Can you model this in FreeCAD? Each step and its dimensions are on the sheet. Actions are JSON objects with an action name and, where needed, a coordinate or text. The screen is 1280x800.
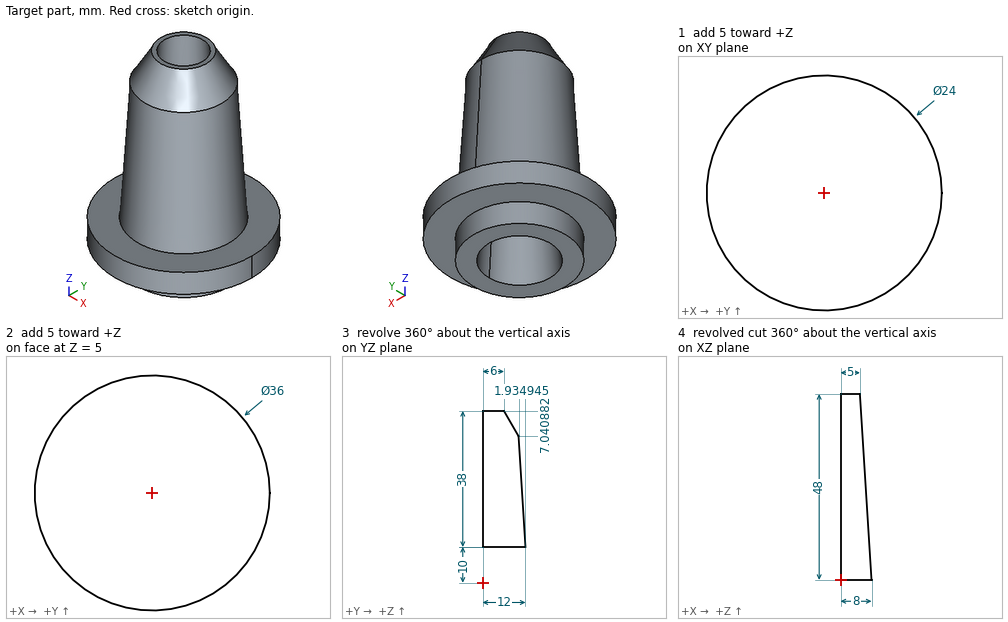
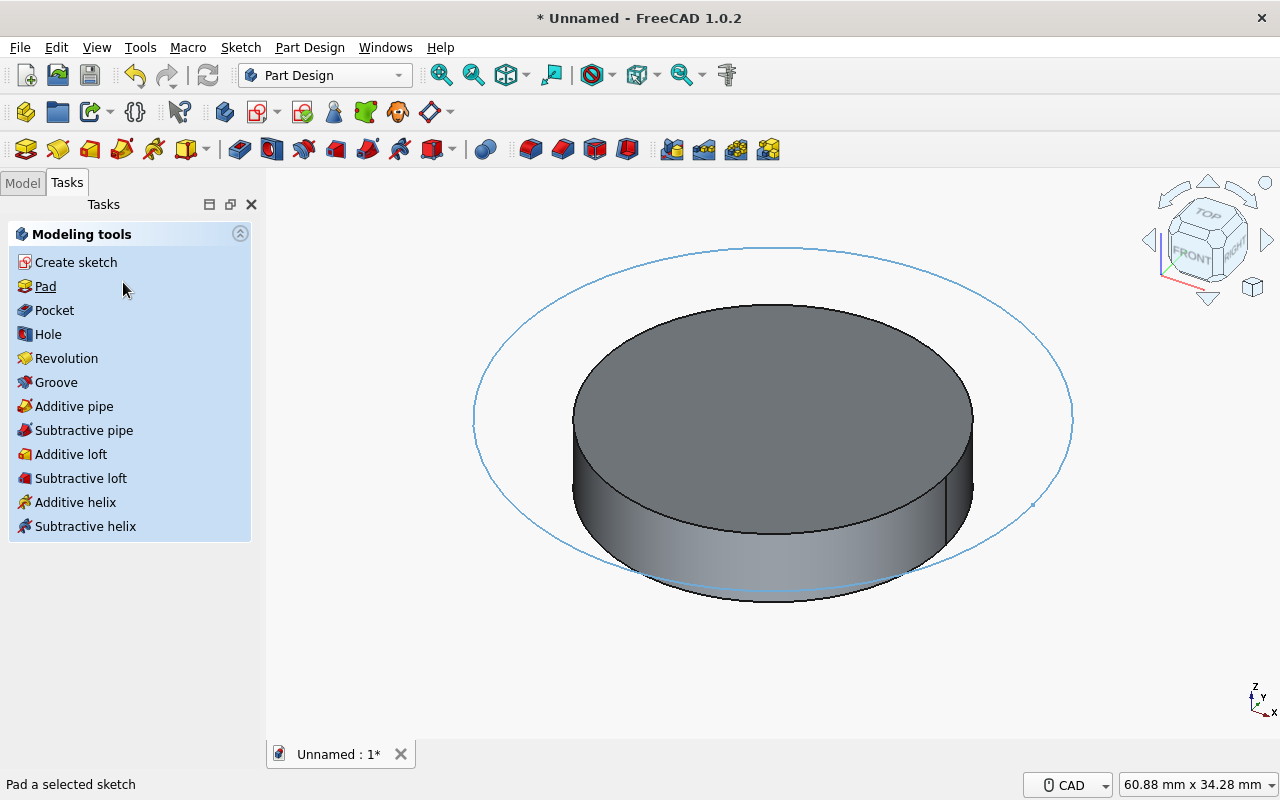
{"action": "left_click", "coordinate": [26, 150]}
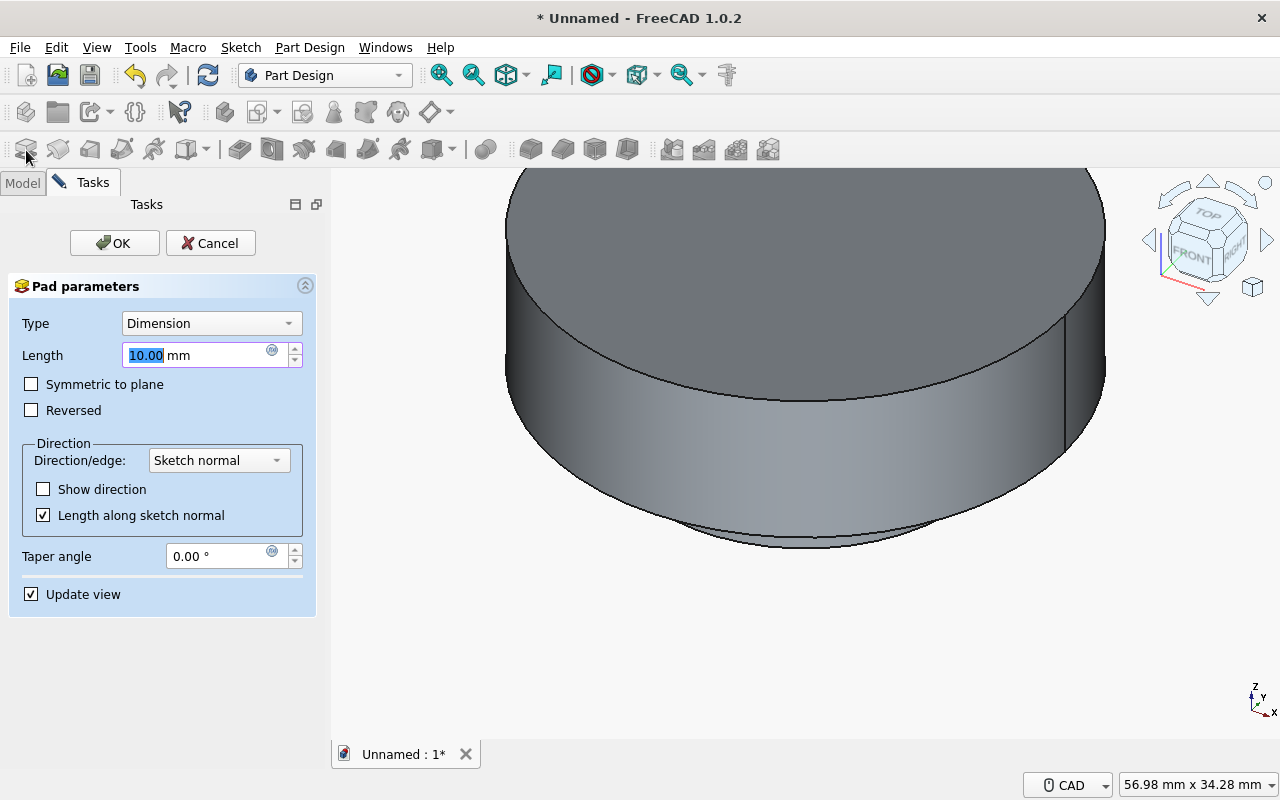
{"action": "type", "text": "5"}
{"action": "key", "text": "Tab"}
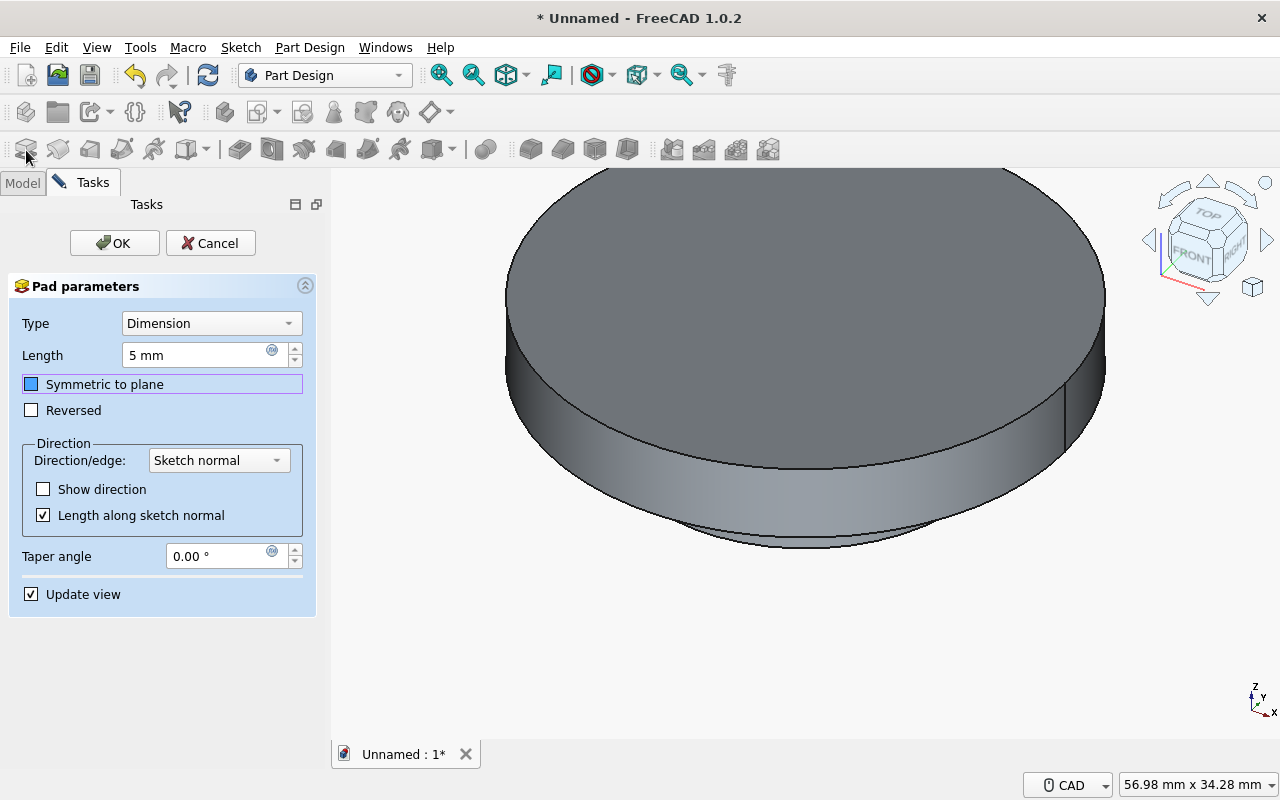
{"action": "left_click", "coordinate": [115, 243]}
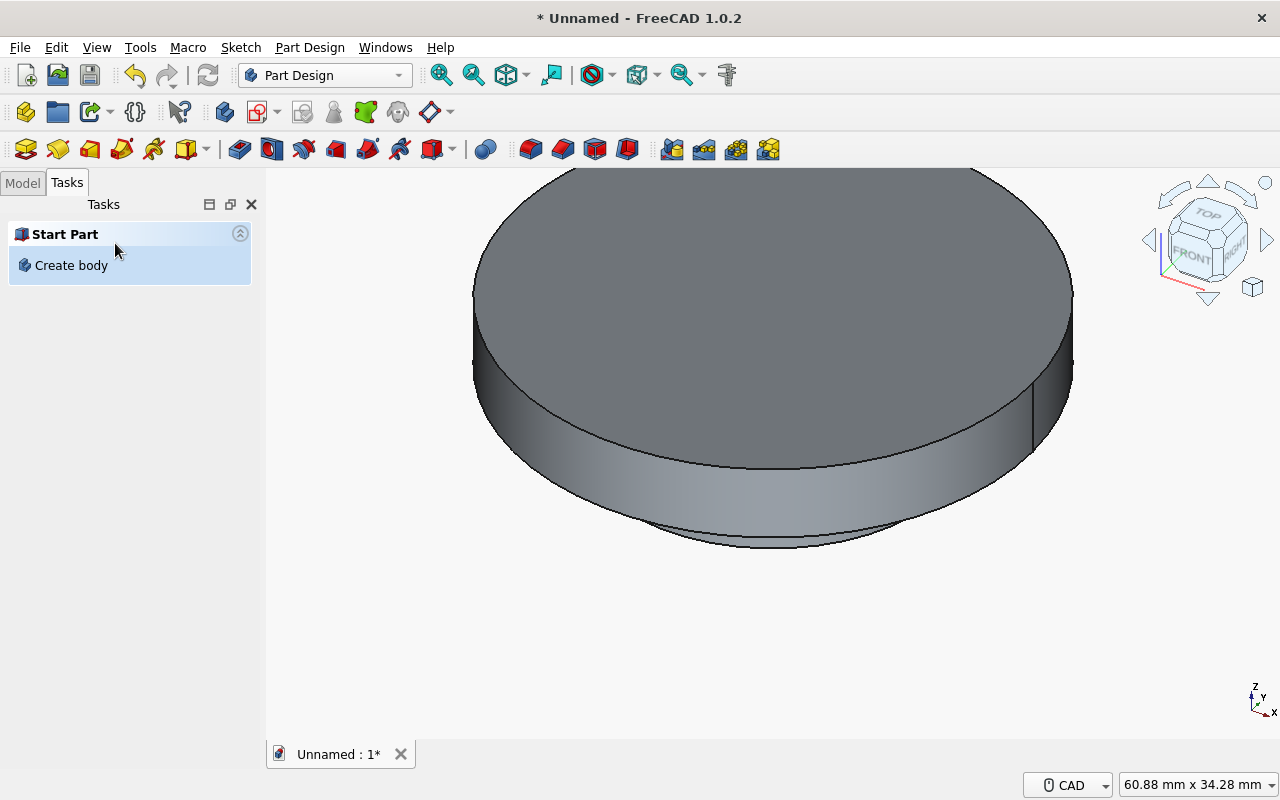
{"action": "left_click", "coordinate": [442, 76]}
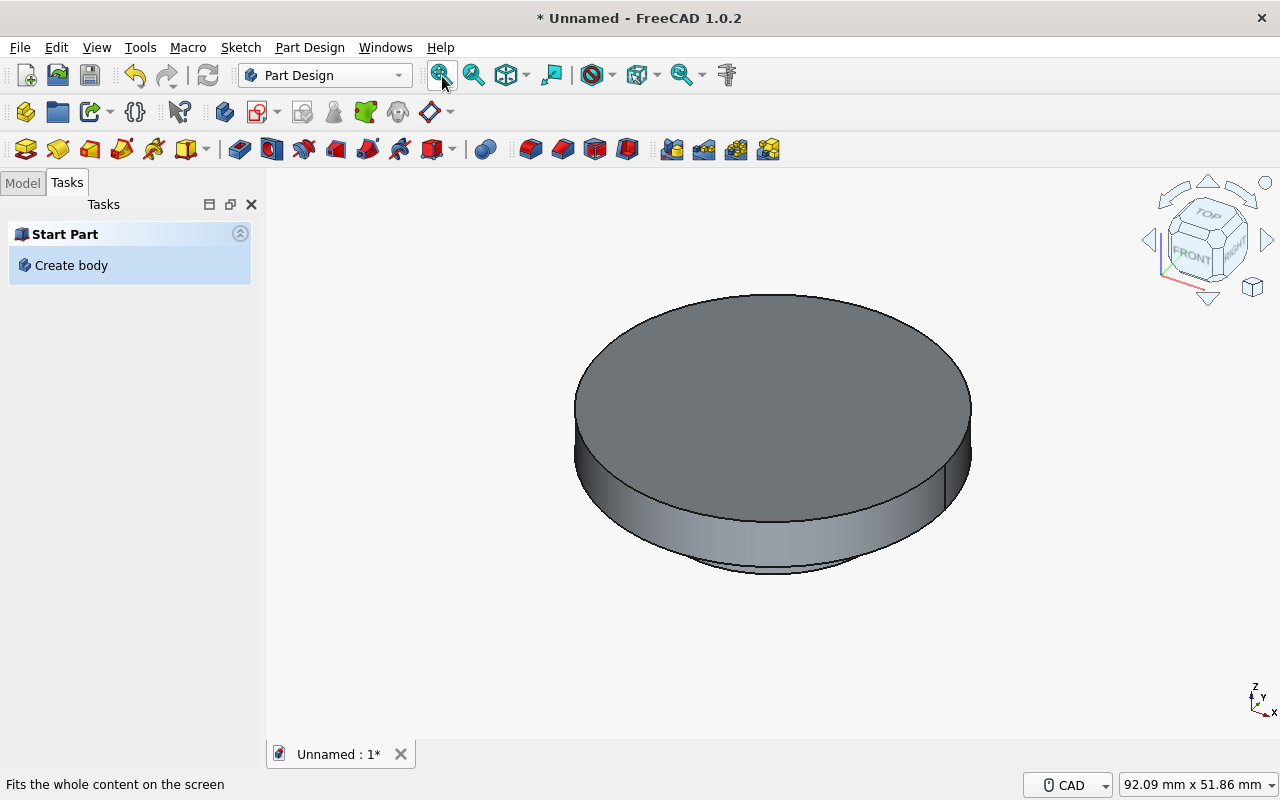
{"action": "left_click", "coordinate": [258, 112]}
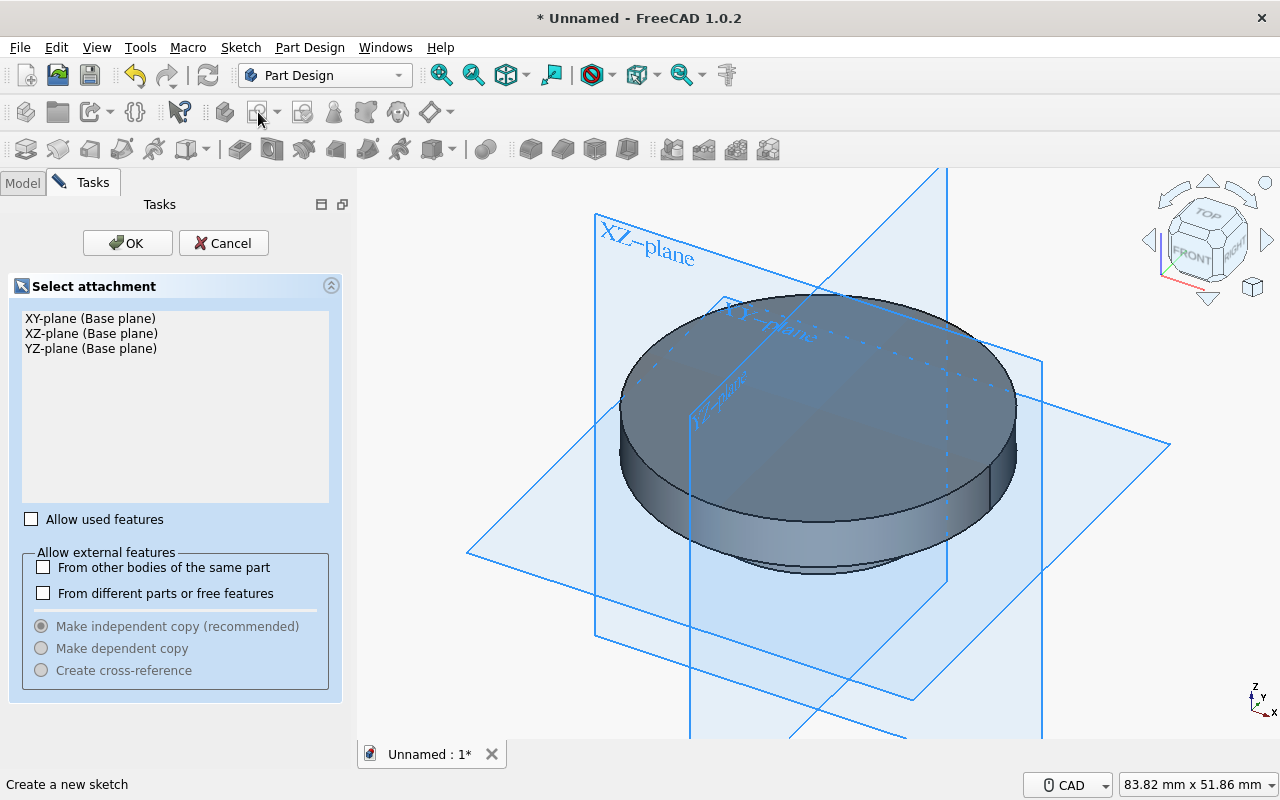
{"action": "left_click", "coordinate": [82, 348]}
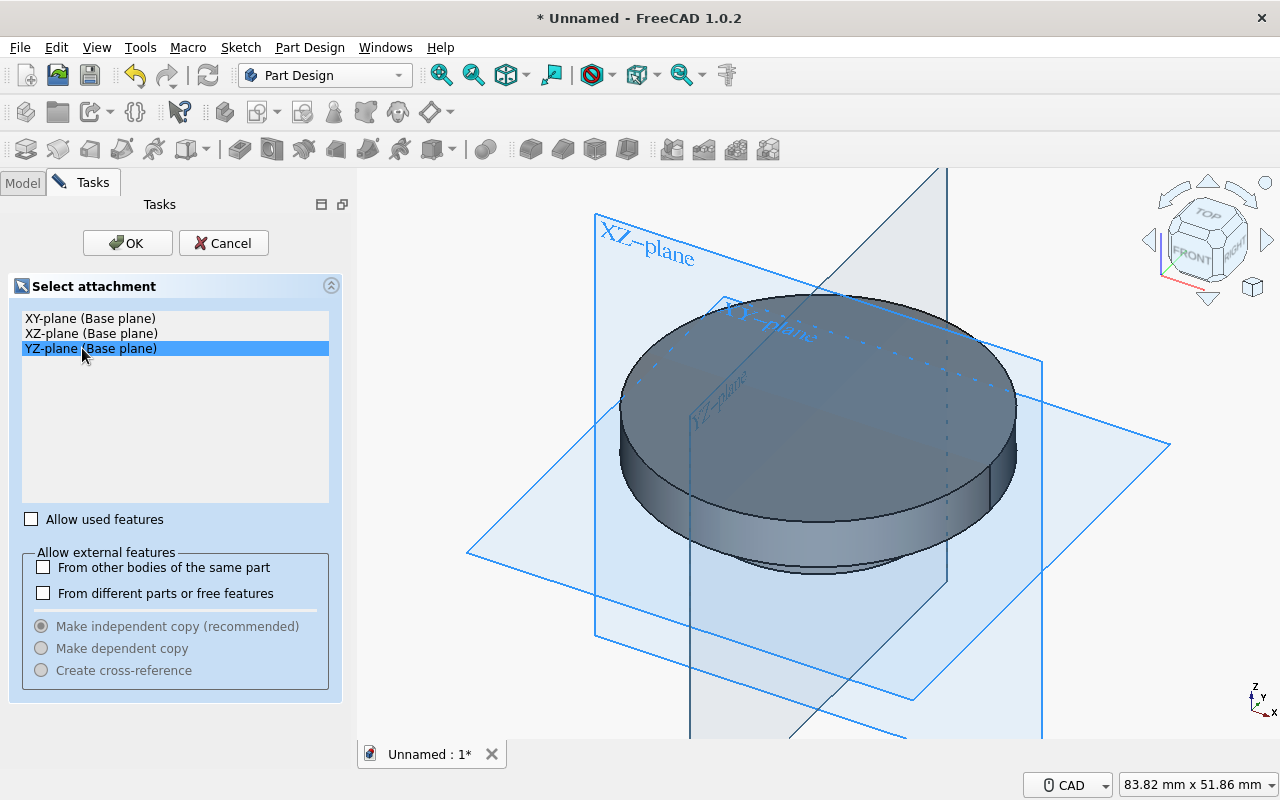
{"action": "left_click", "coordinate": [128, 243]}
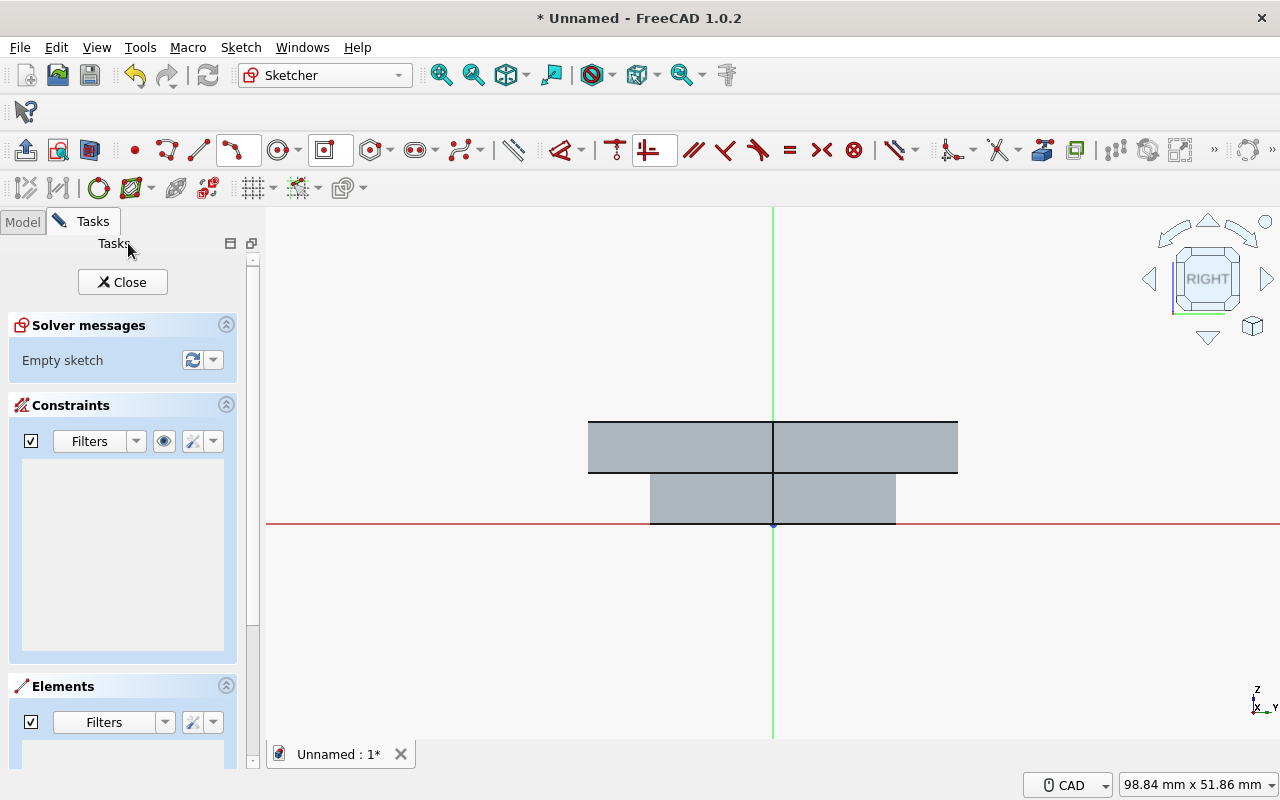
{"action": "left_click", "coordinate": [90, 150]}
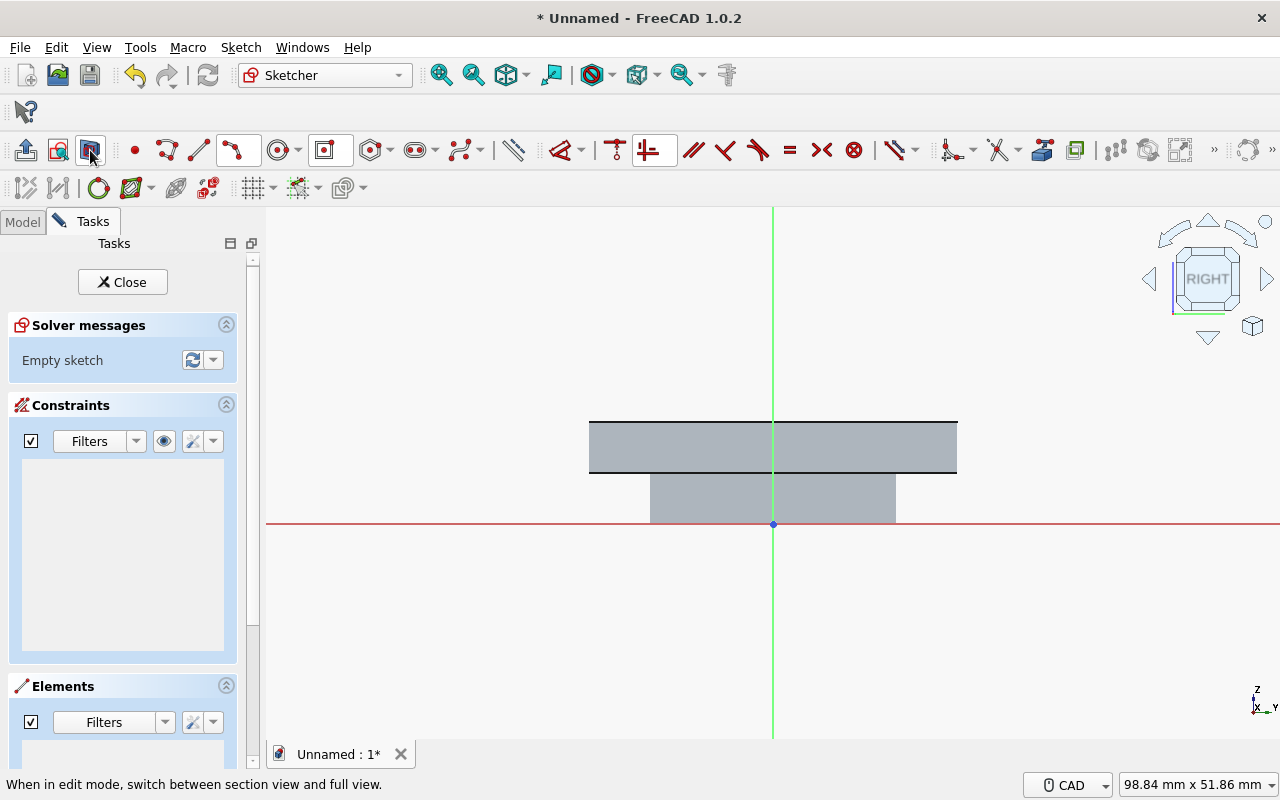
{"action": "scroll", "coordinate": [546, 710], "scroll_direction": "down", "scroll_amount": 3}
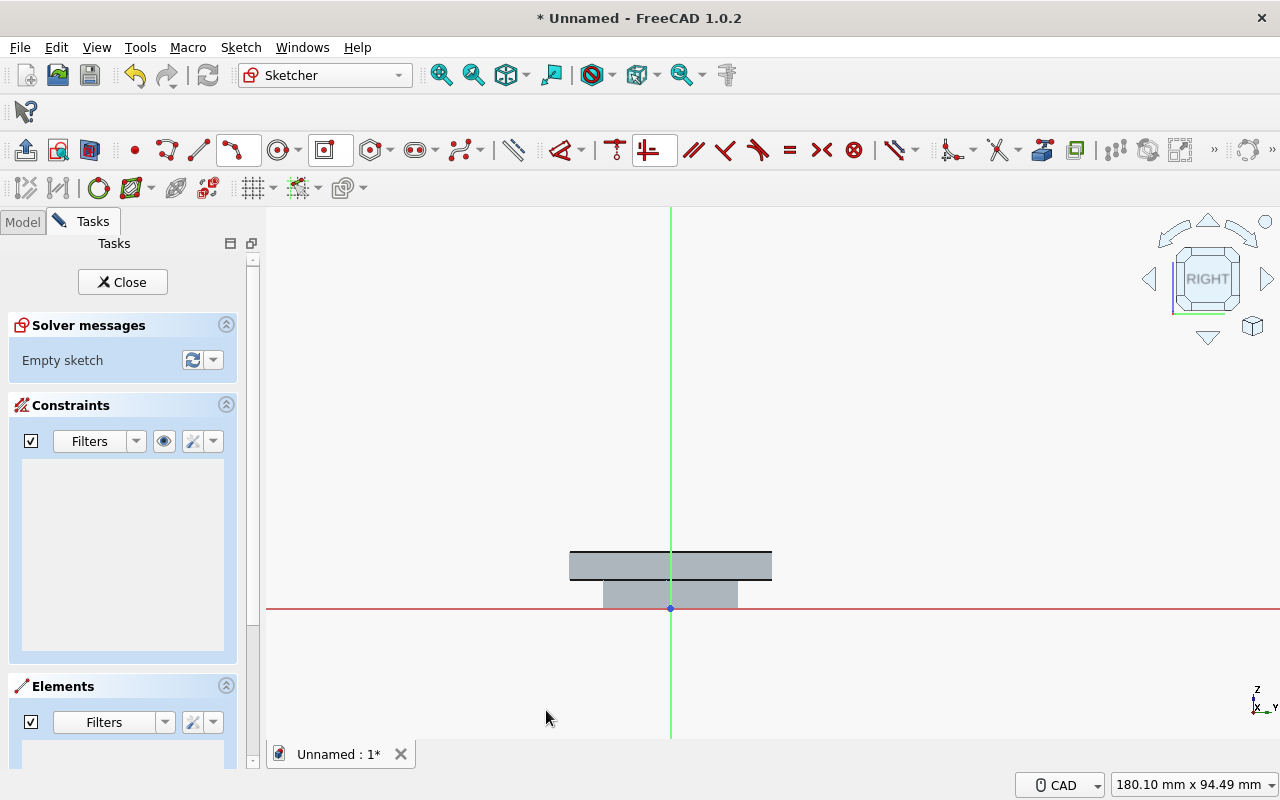
{"action": "left_click", "coordinate": [168, 150]}